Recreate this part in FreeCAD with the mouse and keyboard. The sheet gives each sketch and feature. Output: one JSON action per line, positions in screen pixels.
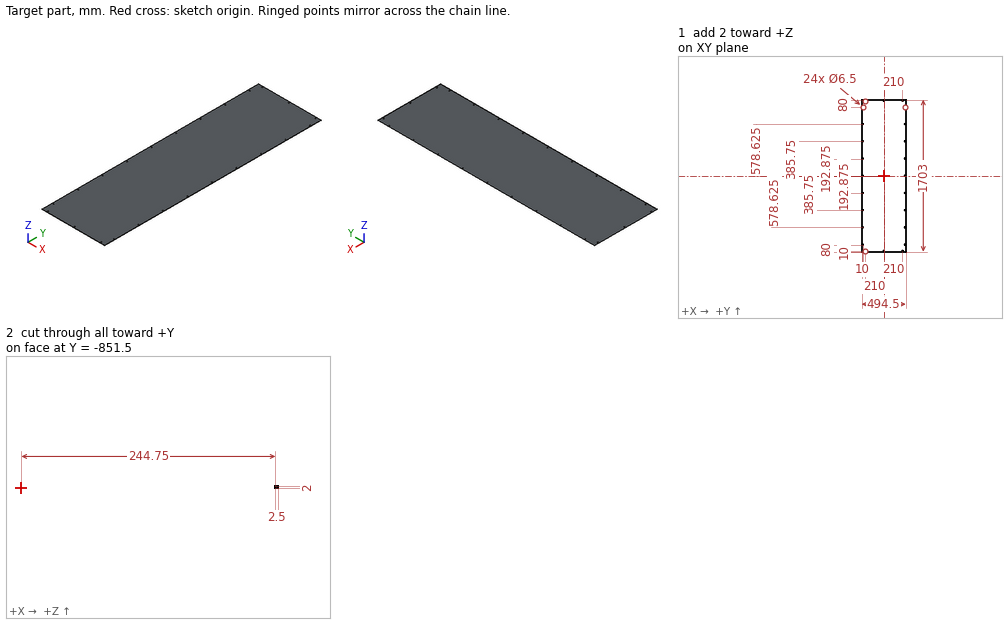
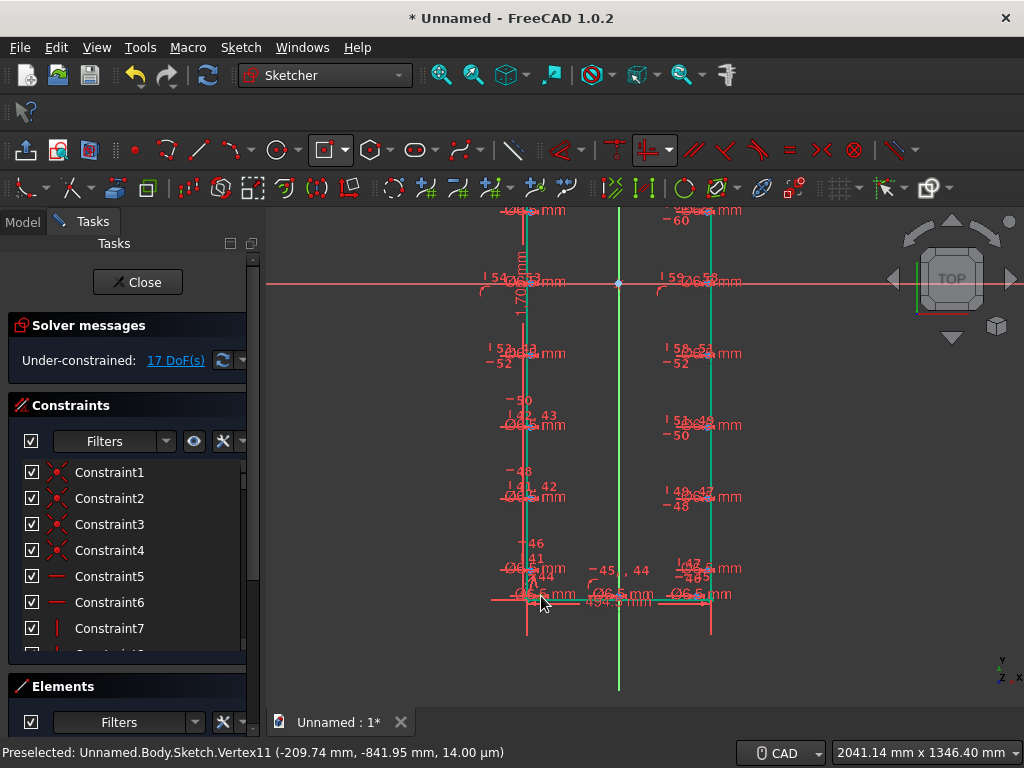
{"action": "scroll", "coordinate": [542, 598], "scroll_direction": "down", "scroll_amount": 4}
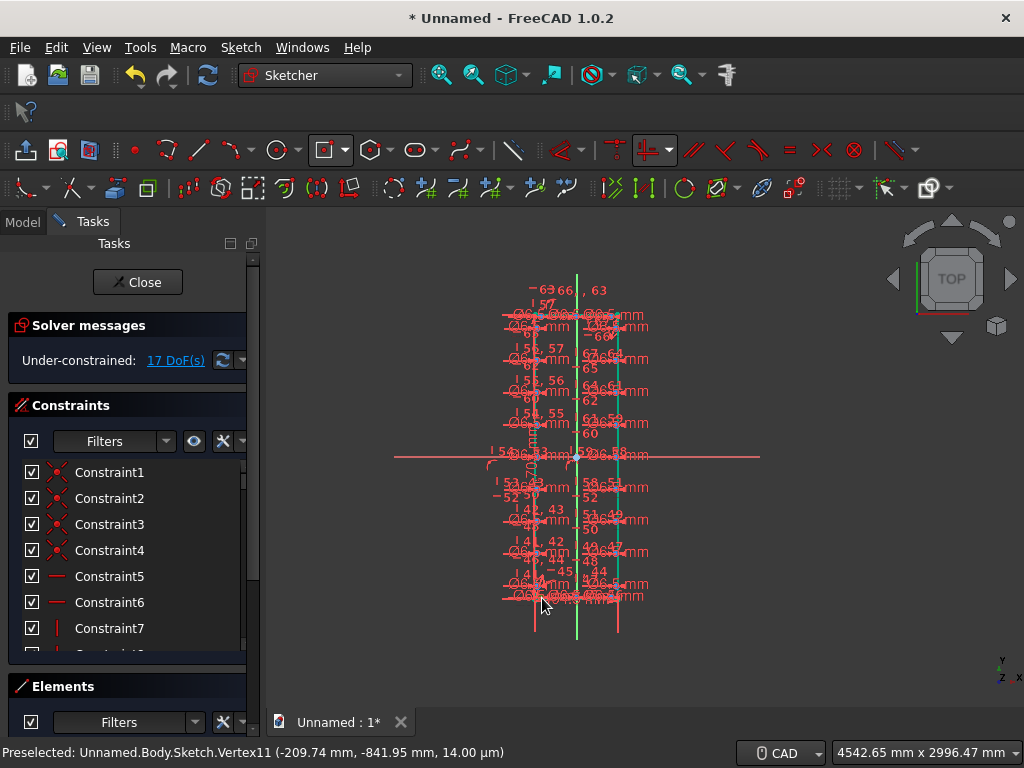
{"action": "scroll", "coordinate": [542, 317], "scroll_direction": "up", "scroll_amount": 4}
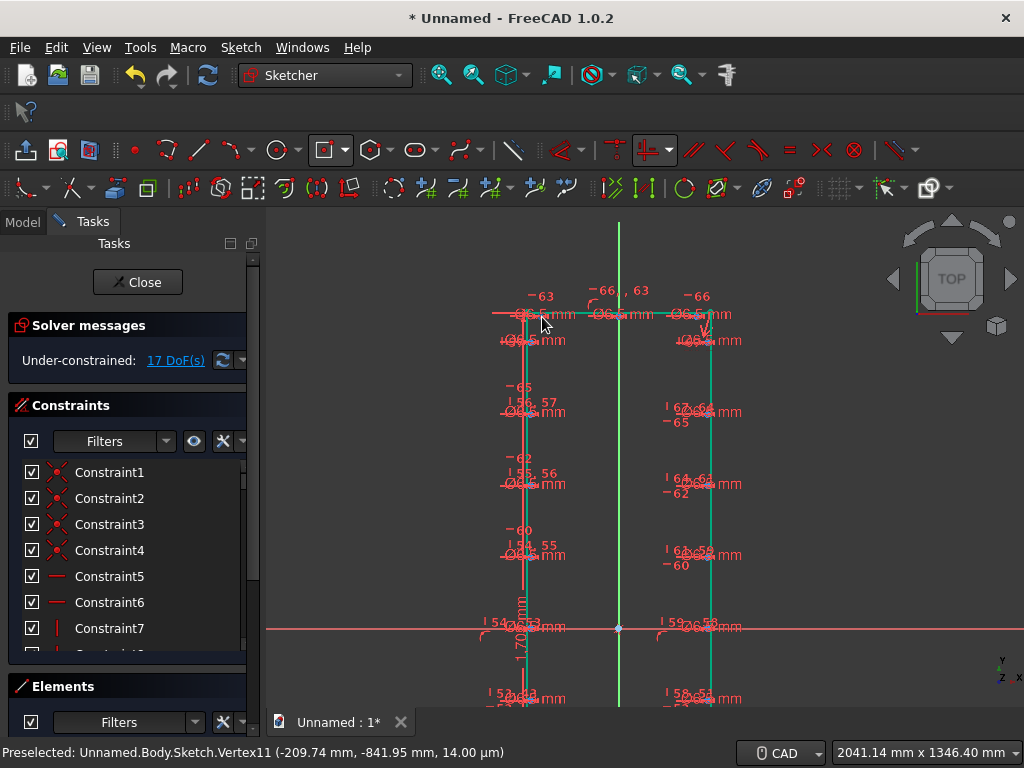
{"action": "left_click", "coordinate": [541, 316]}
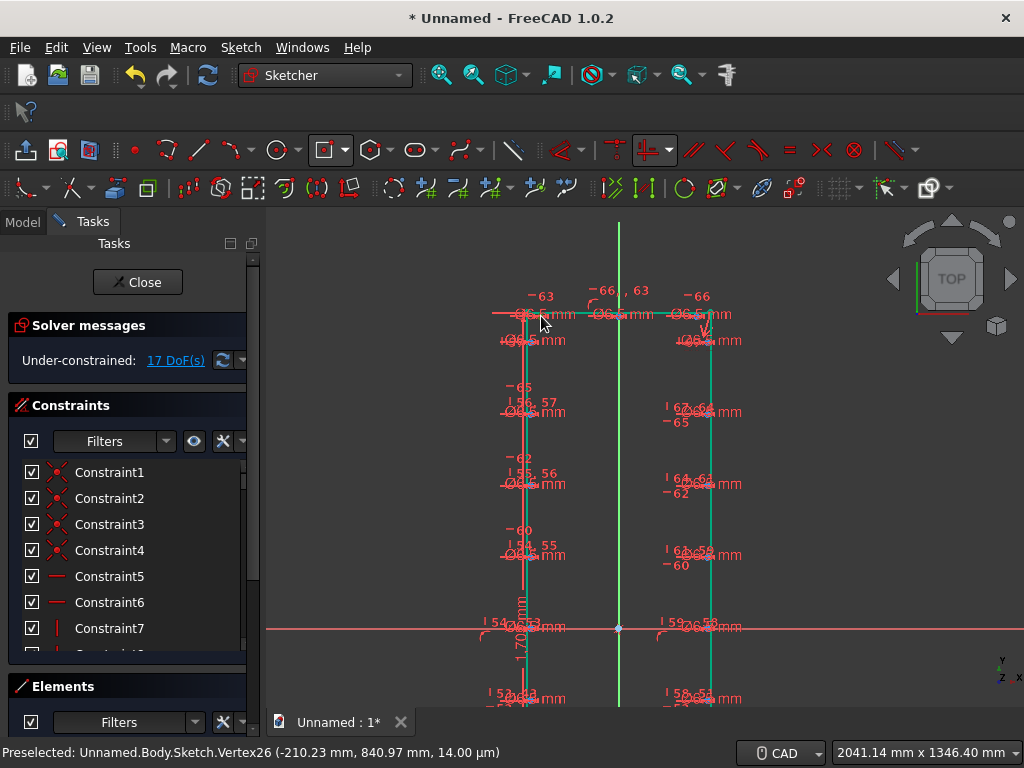
{"action": "left_click", "coordinate": [334, 629]}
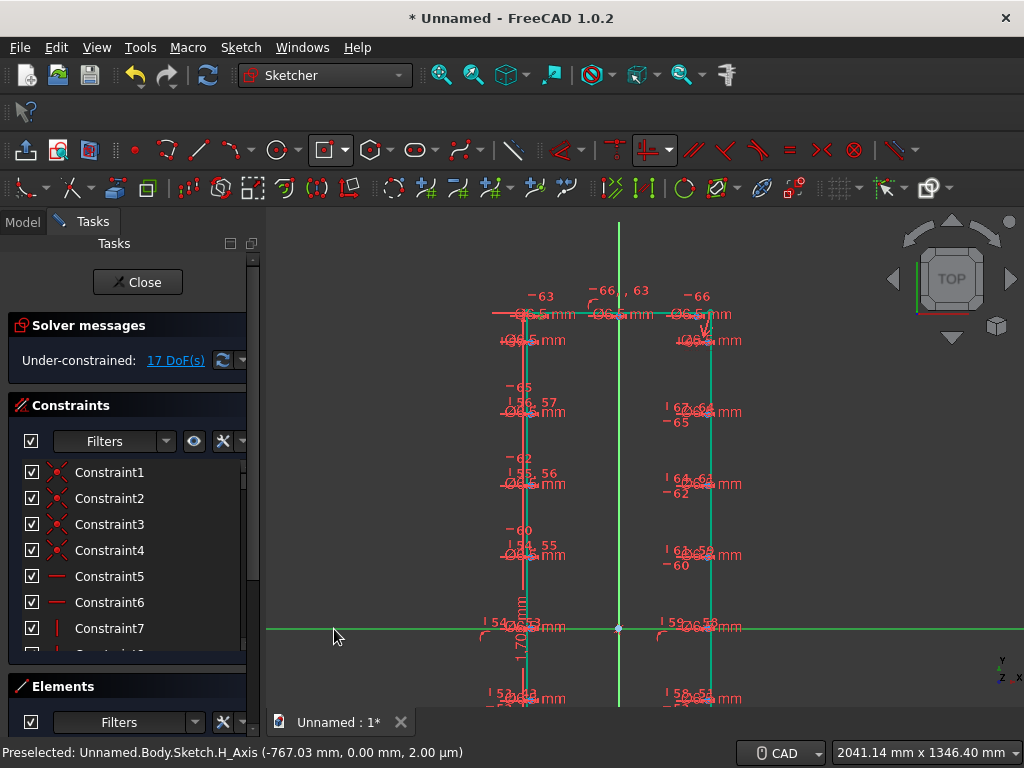
{"action": "left_click", "coordinate": [822, 150]}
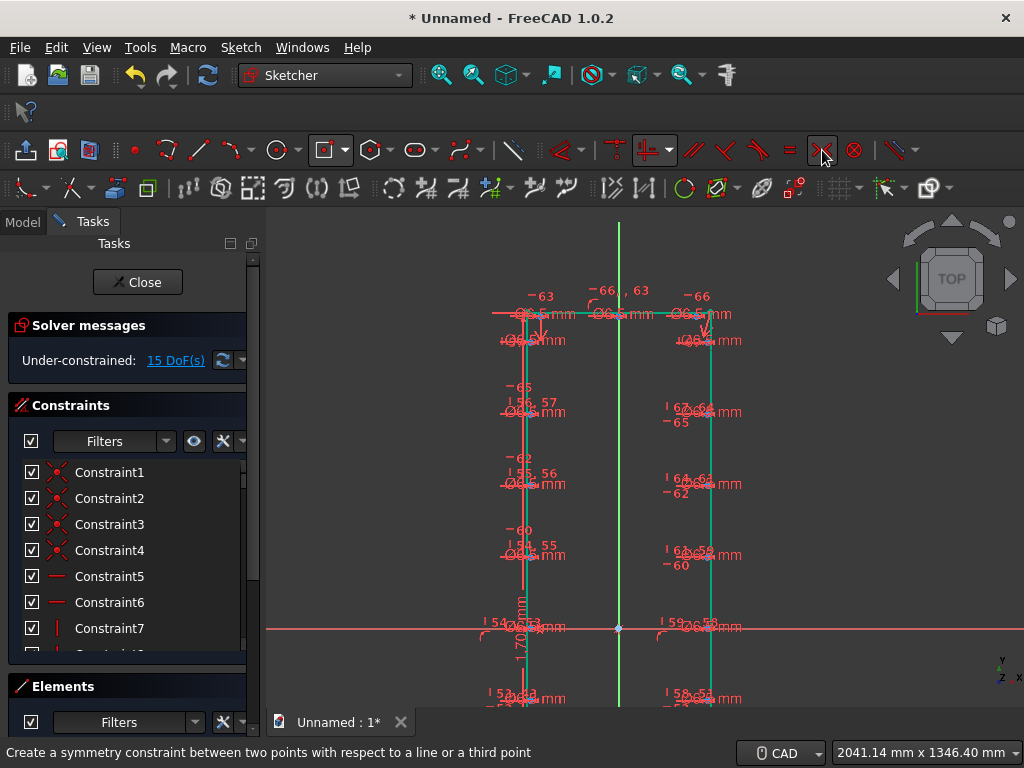
{"action": "left_click", "coordinate": [531, 342]}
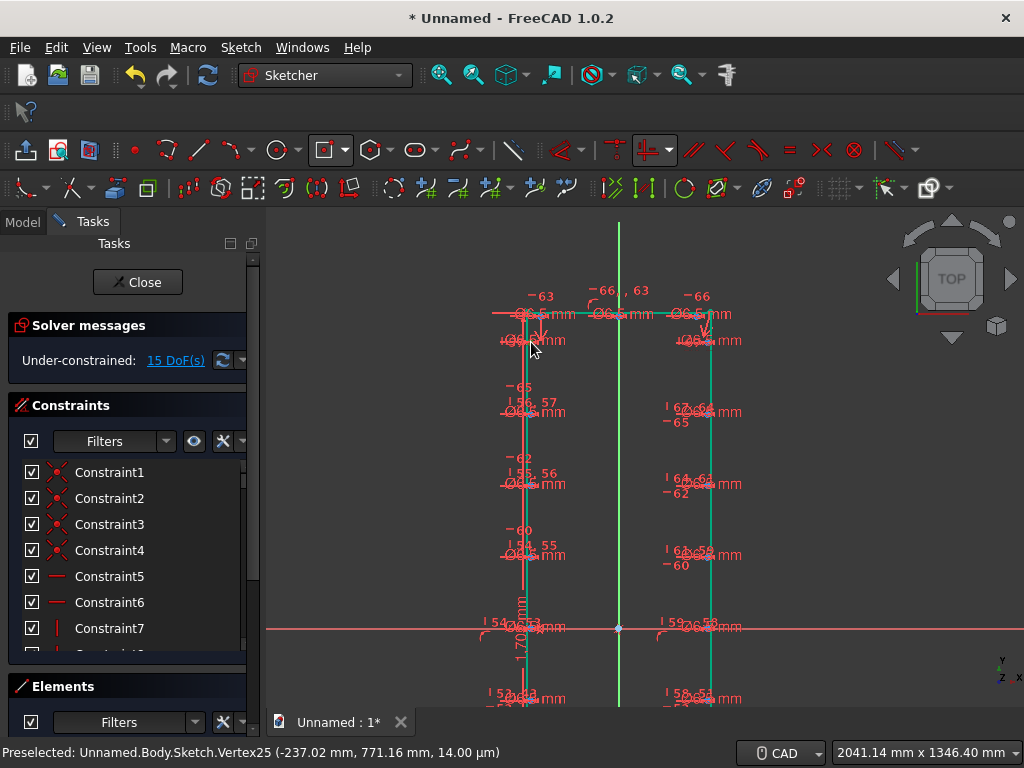
{"action": "left_click", "coordinate": [707, 343]}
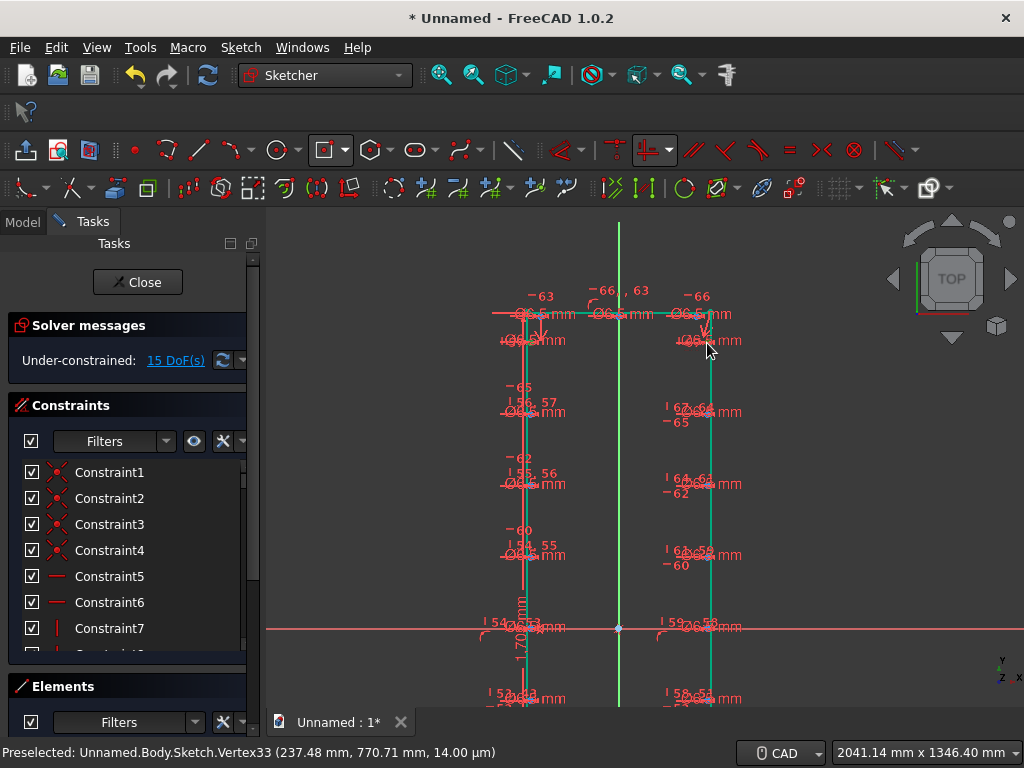
{"action": "left_click", "coordinate": [619, 584]}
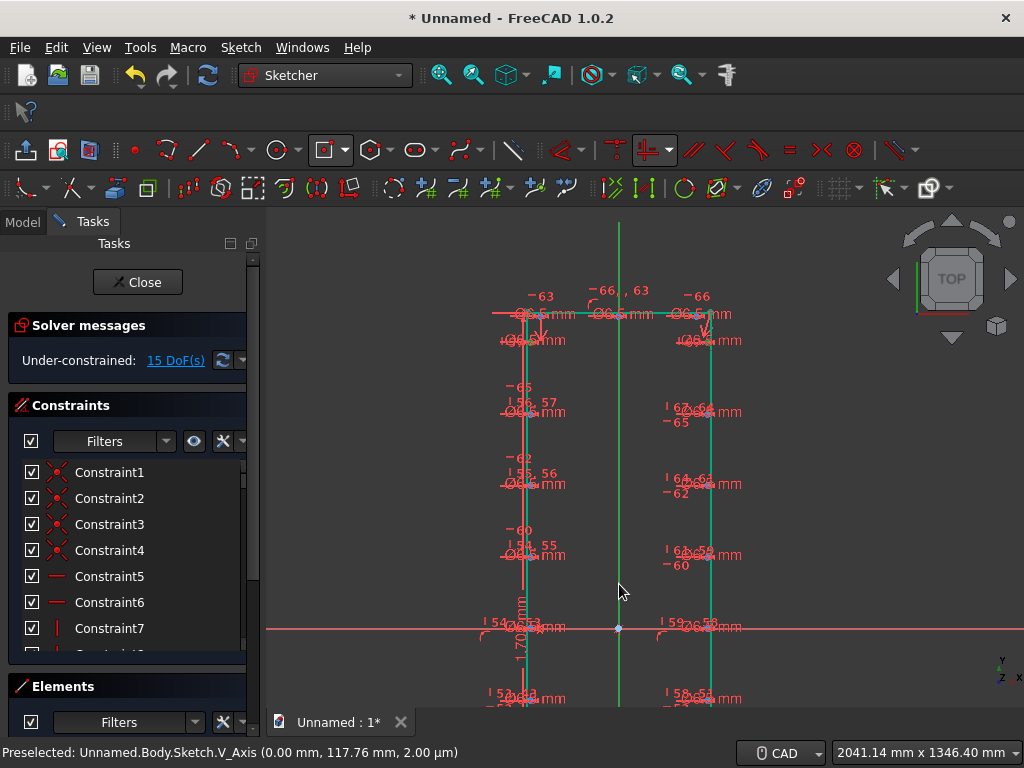
{"action": "left_click", "coordinate": [822, 150]}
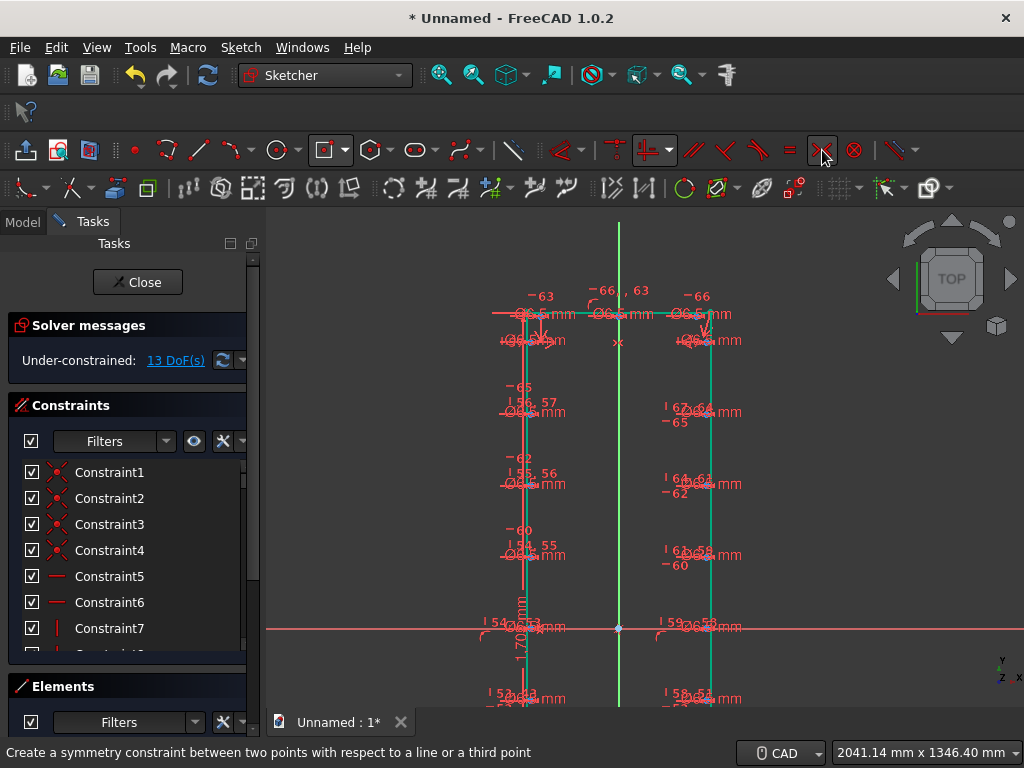
{"action": "scroll", "coordinate": [542, 317], "scroll_direction": "down", "scroll_amount": 4}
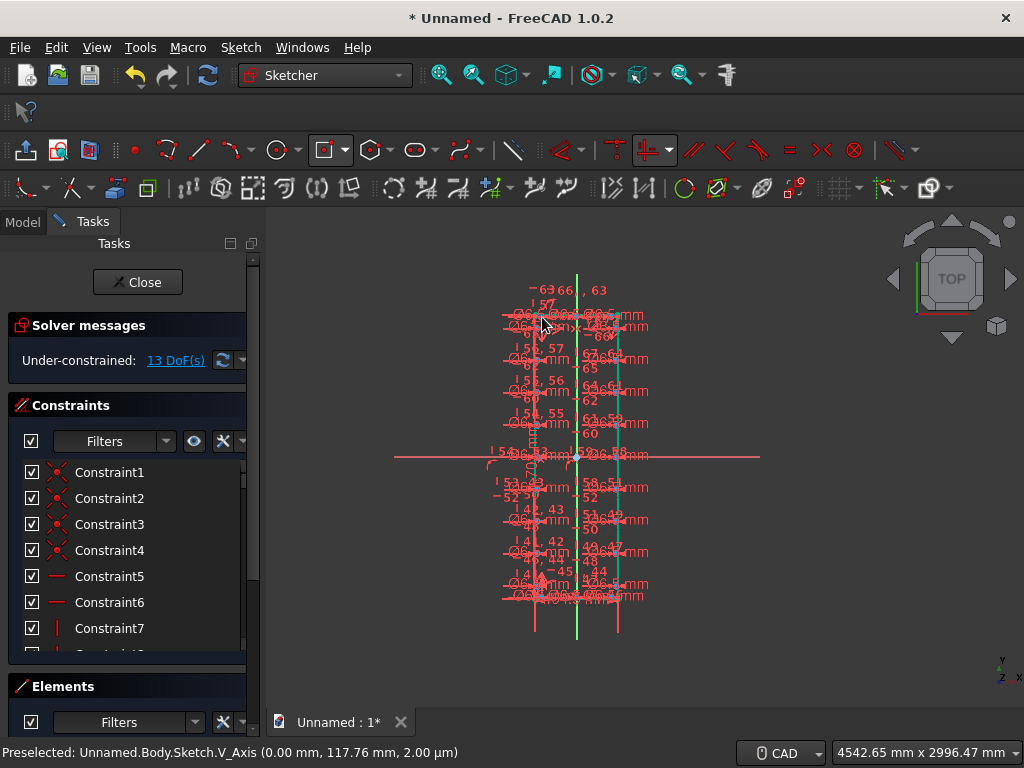
{"action": "scroll", "coordinate": [542, 598], "scroll_direction": "up", "scroll_amount": 4}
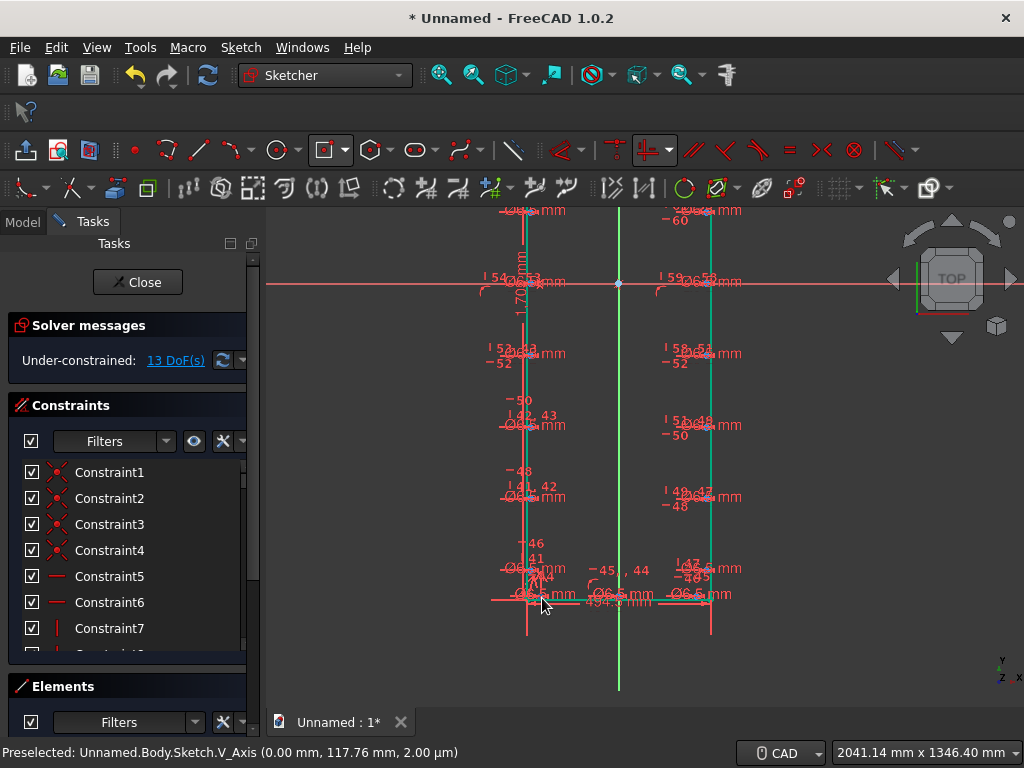
{"action": "left_click", "coordinate": [541, 596]}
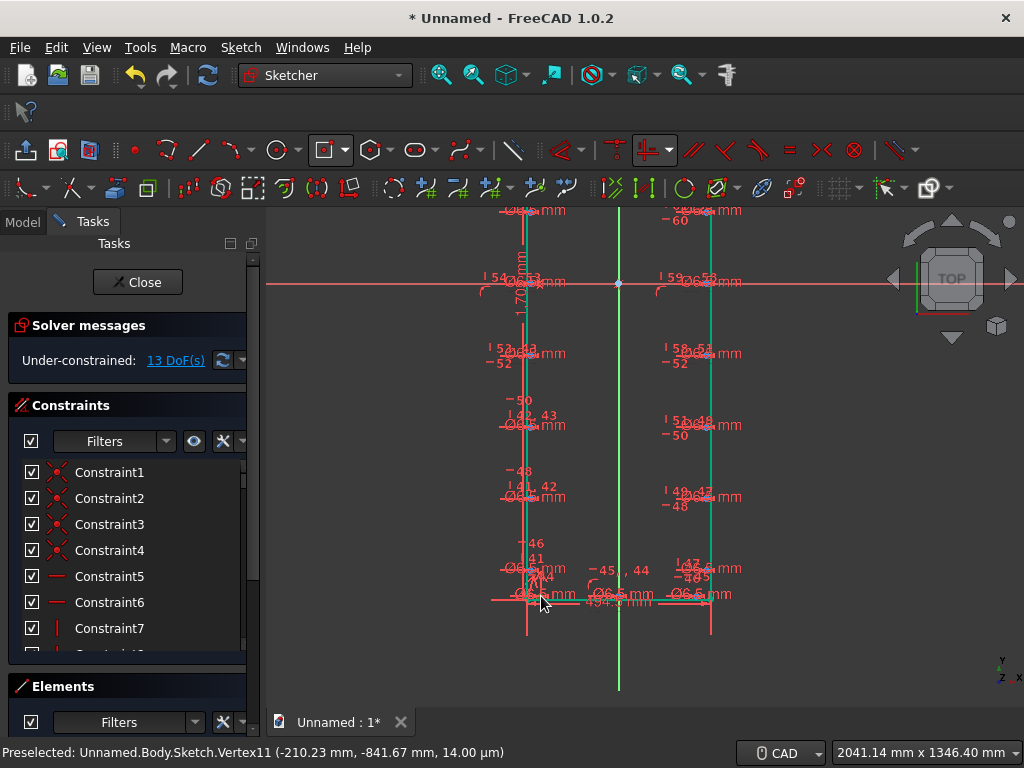
{"action": "left_click", "coordinate": [584, 150]}